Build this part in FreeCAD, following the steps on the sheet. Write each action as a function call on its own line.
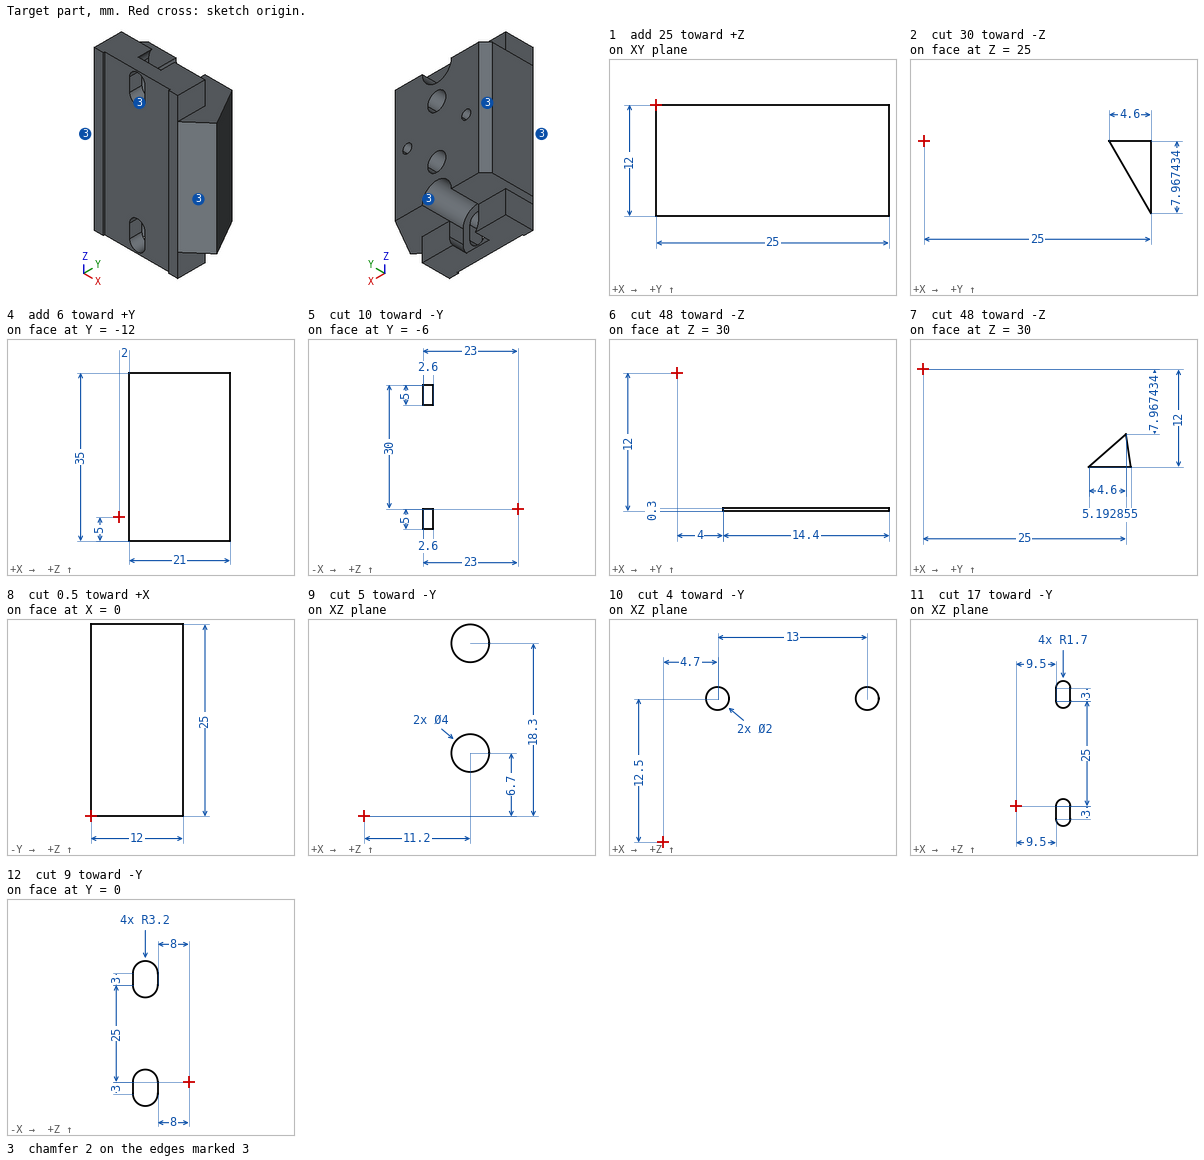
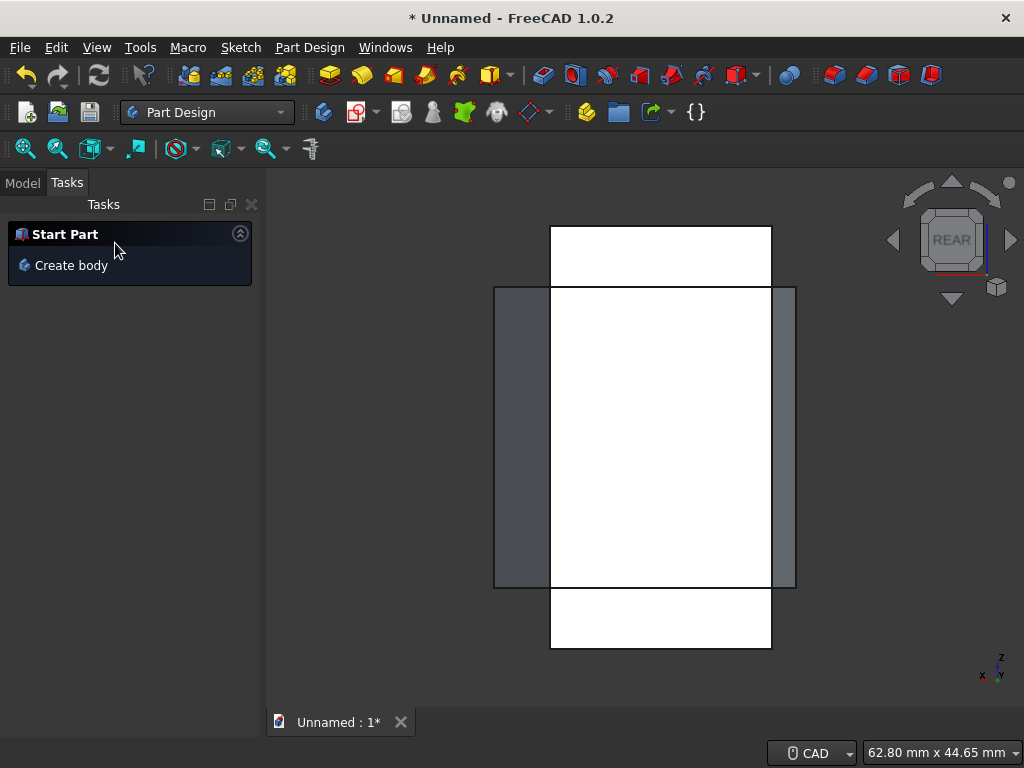
key(0)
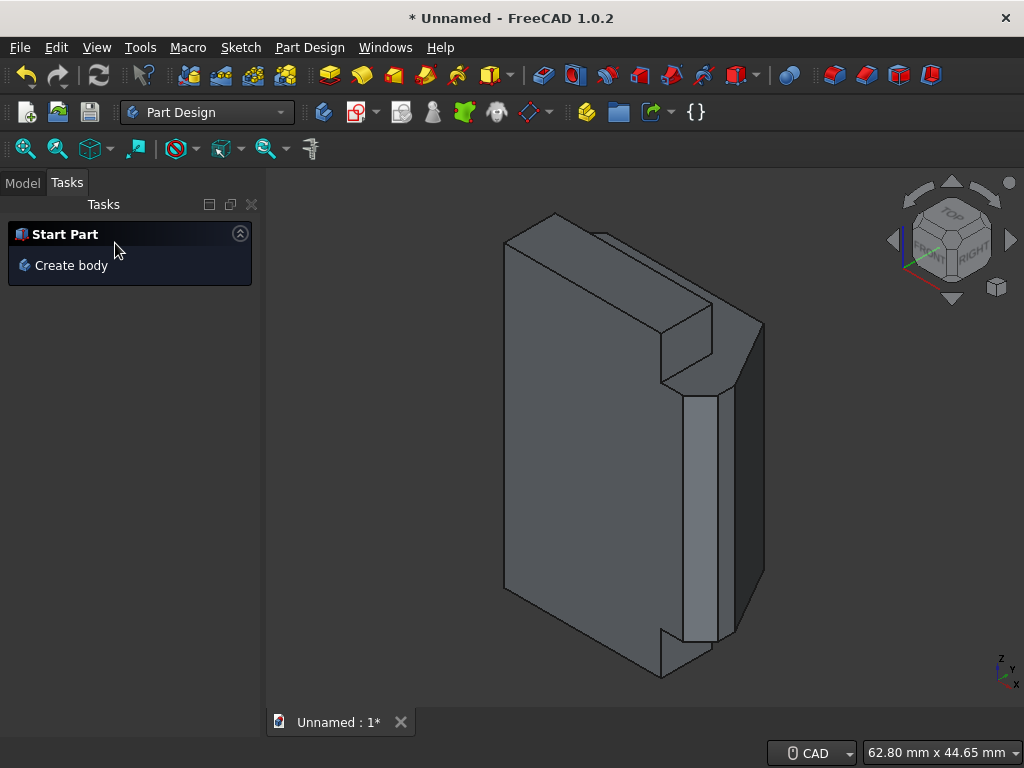
click(653, 298)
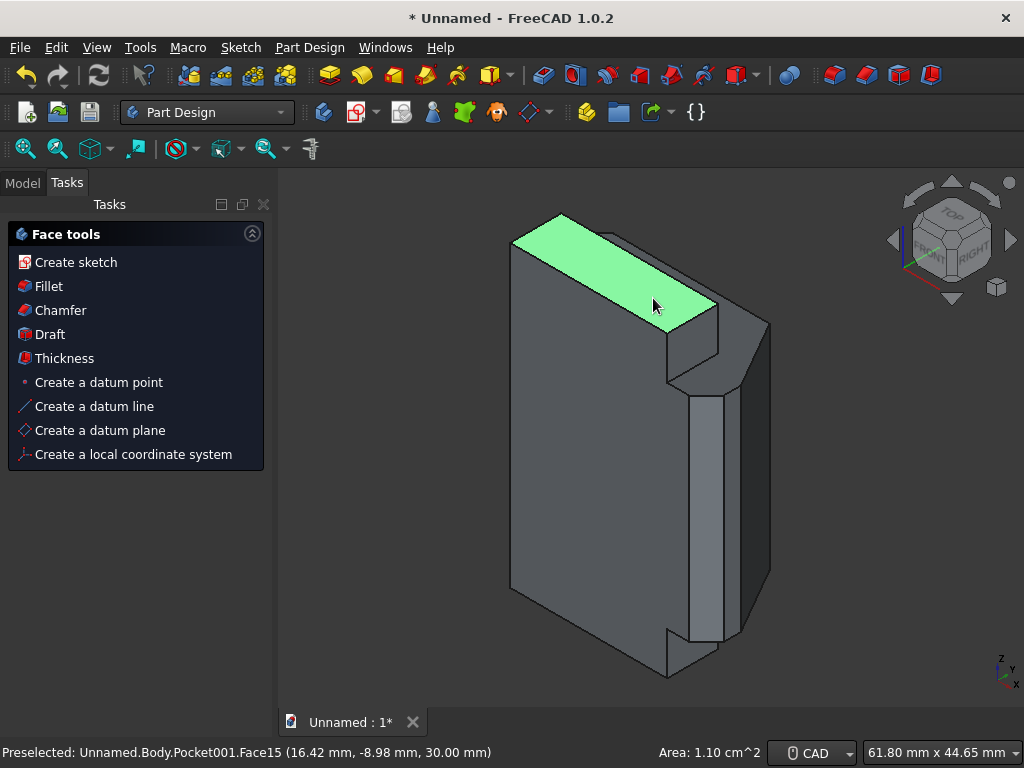
click(356, 112)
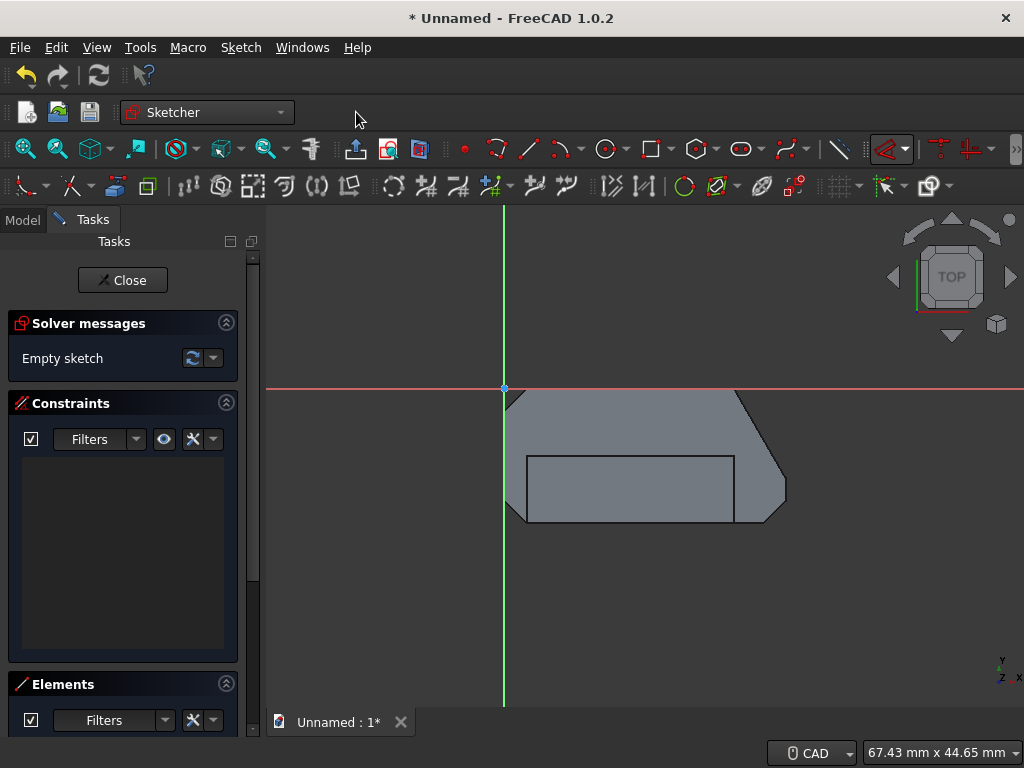
scroll(646, 456, up, 3)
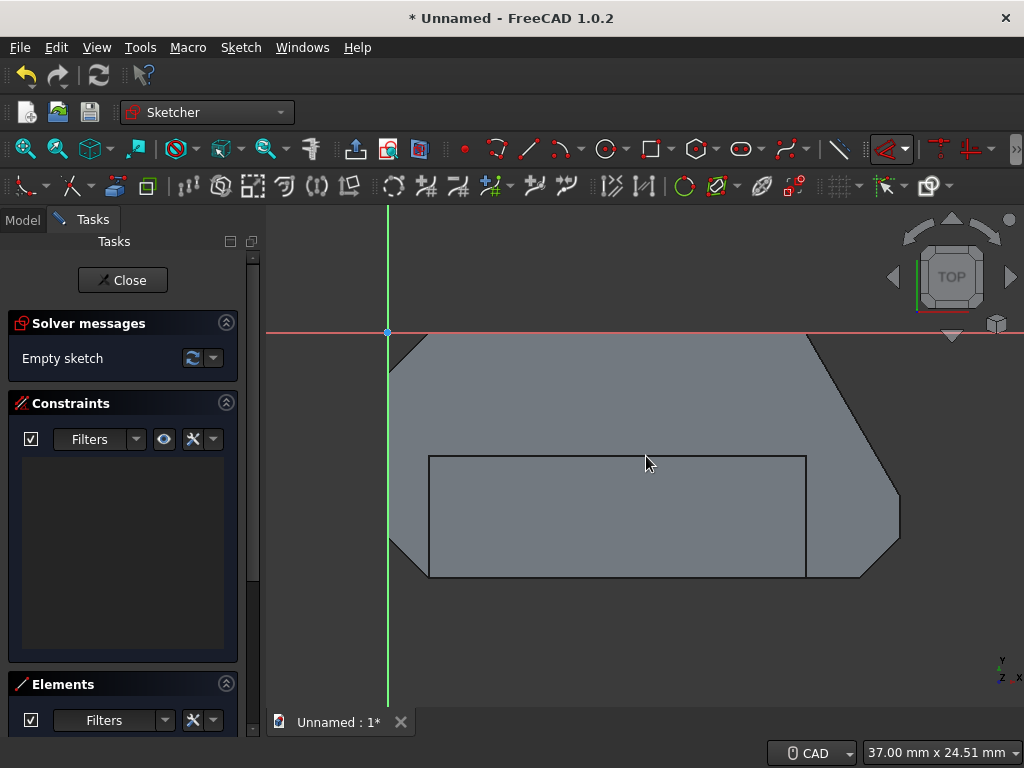
click(652, 150)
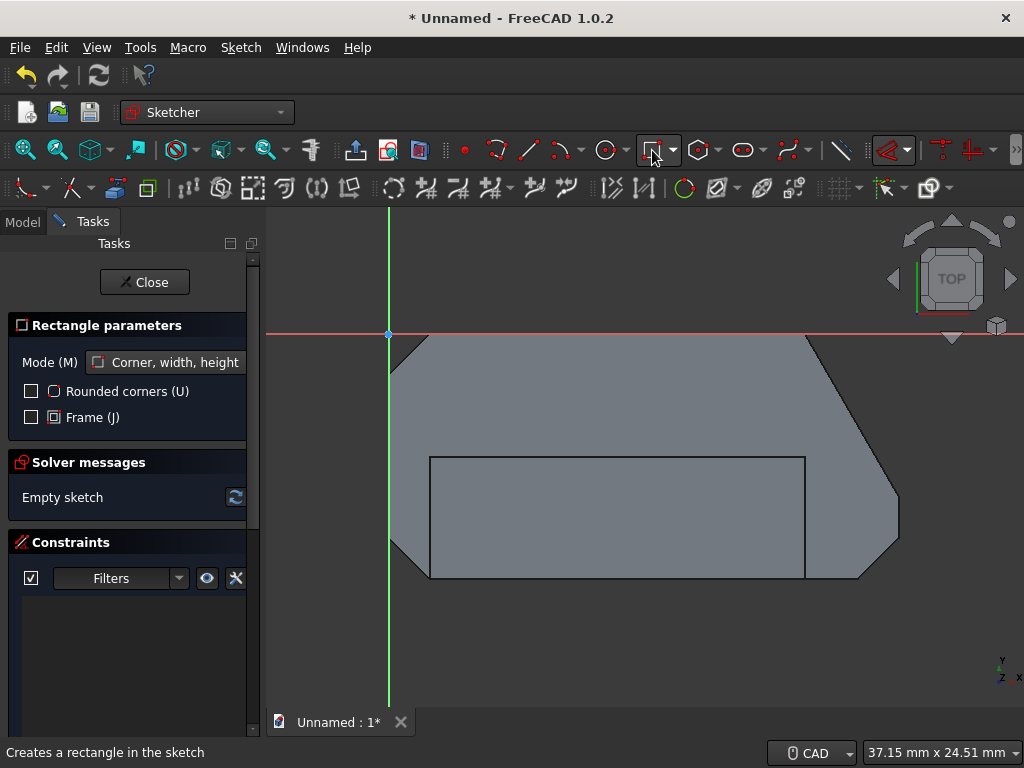
scroll(470, 573, up, 5)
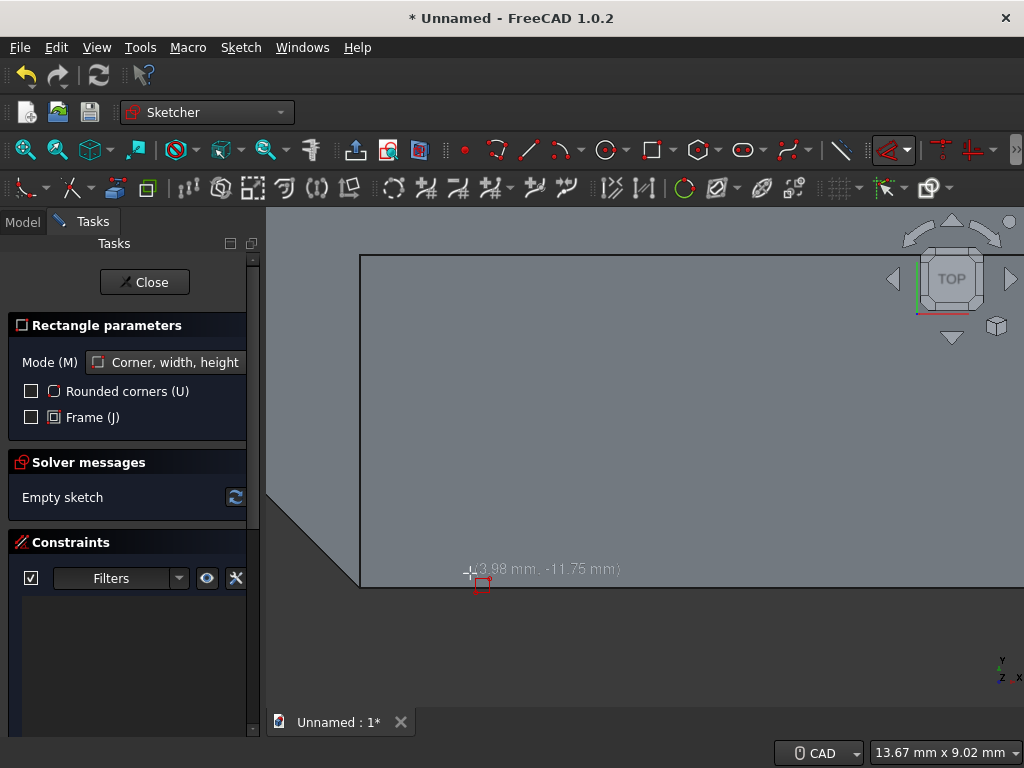
click(470, 571)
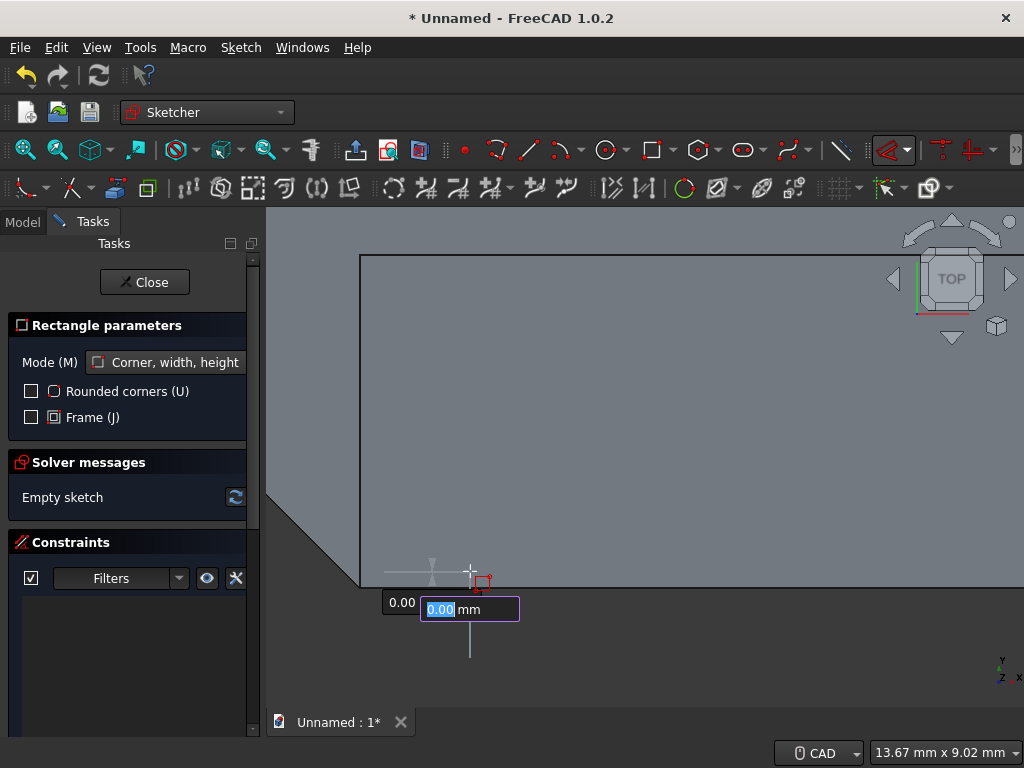
scroll(470, 574, down, 5)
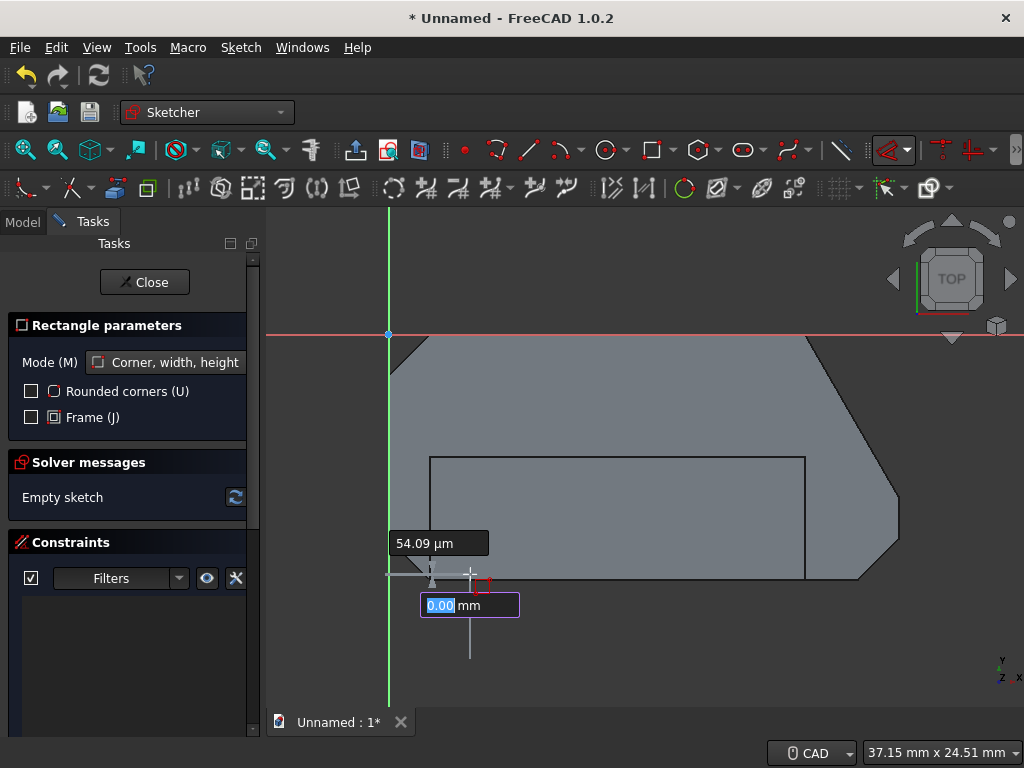
click(764, 580)
key(Escape)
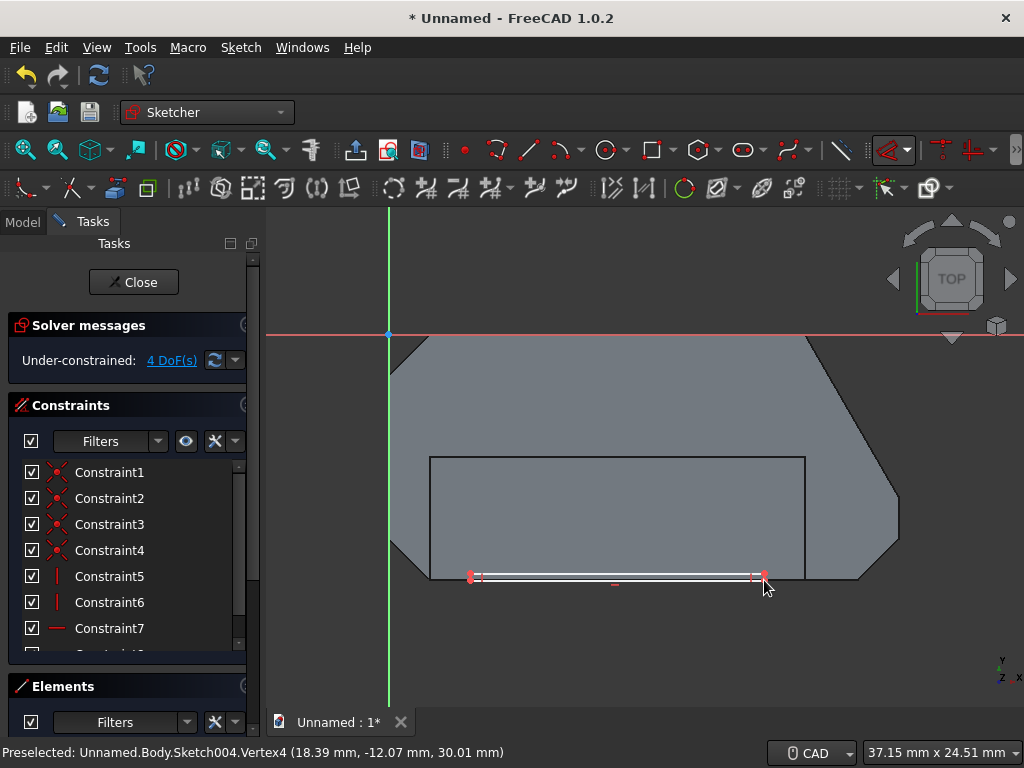
scroll(470, 574, up, 3)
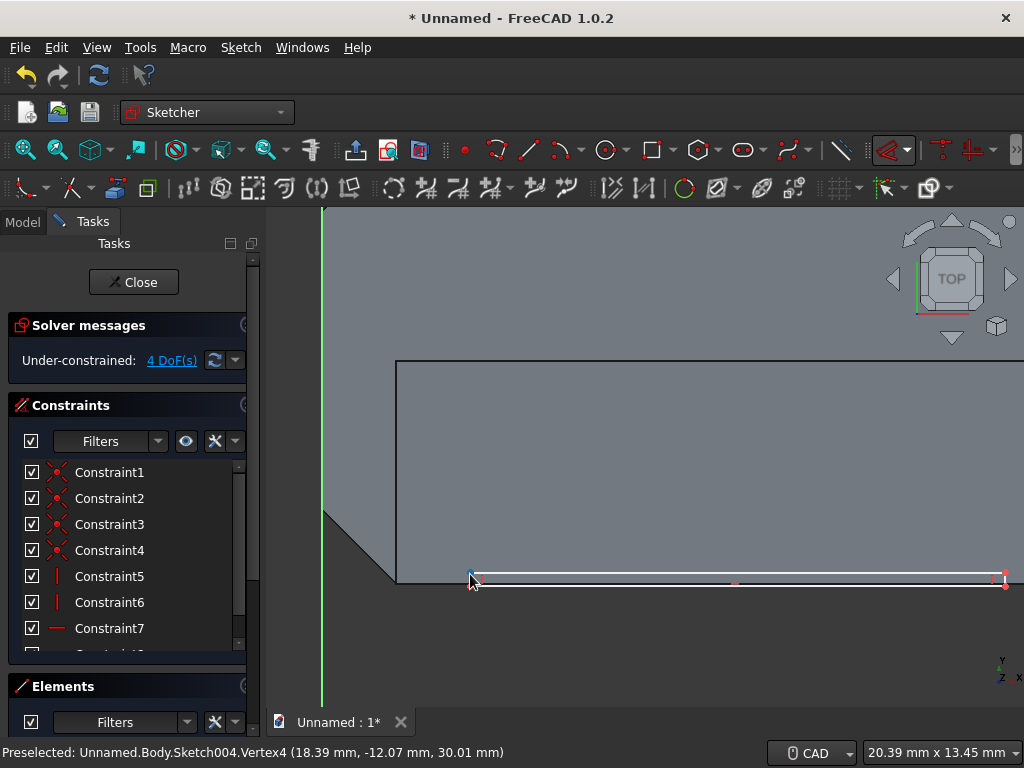
click(470, 573)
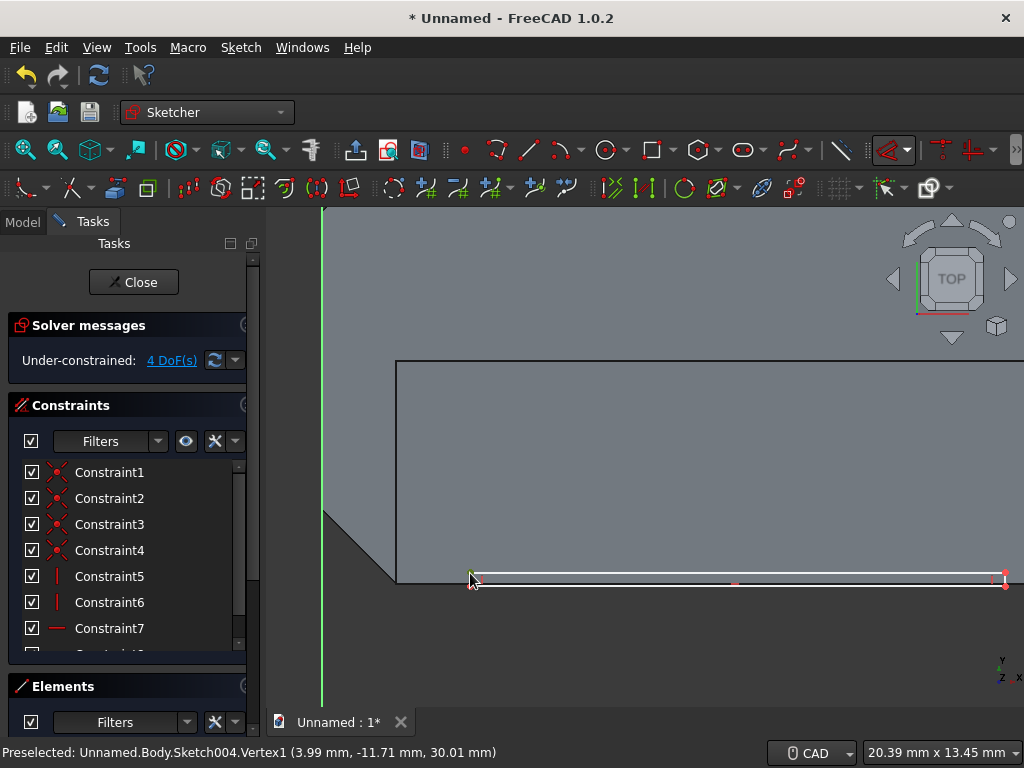
key(l)